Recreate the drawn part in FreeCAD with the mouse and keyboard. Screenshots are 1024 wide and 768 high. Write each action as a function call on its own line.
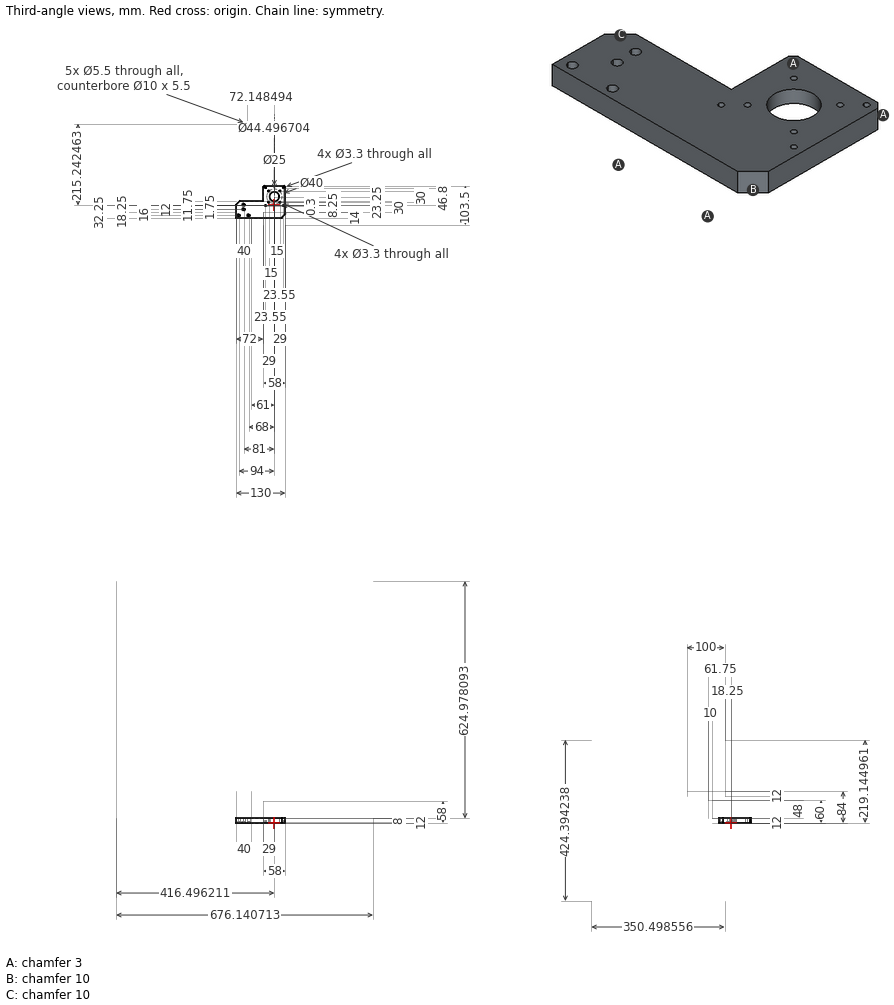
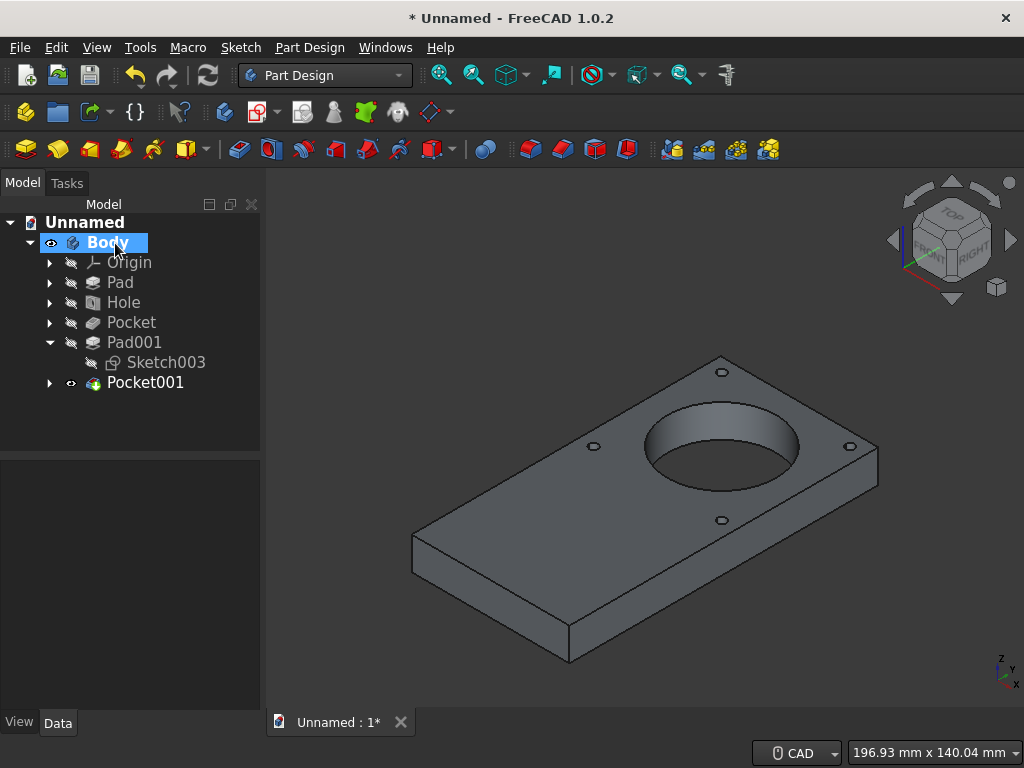
click(569, 644)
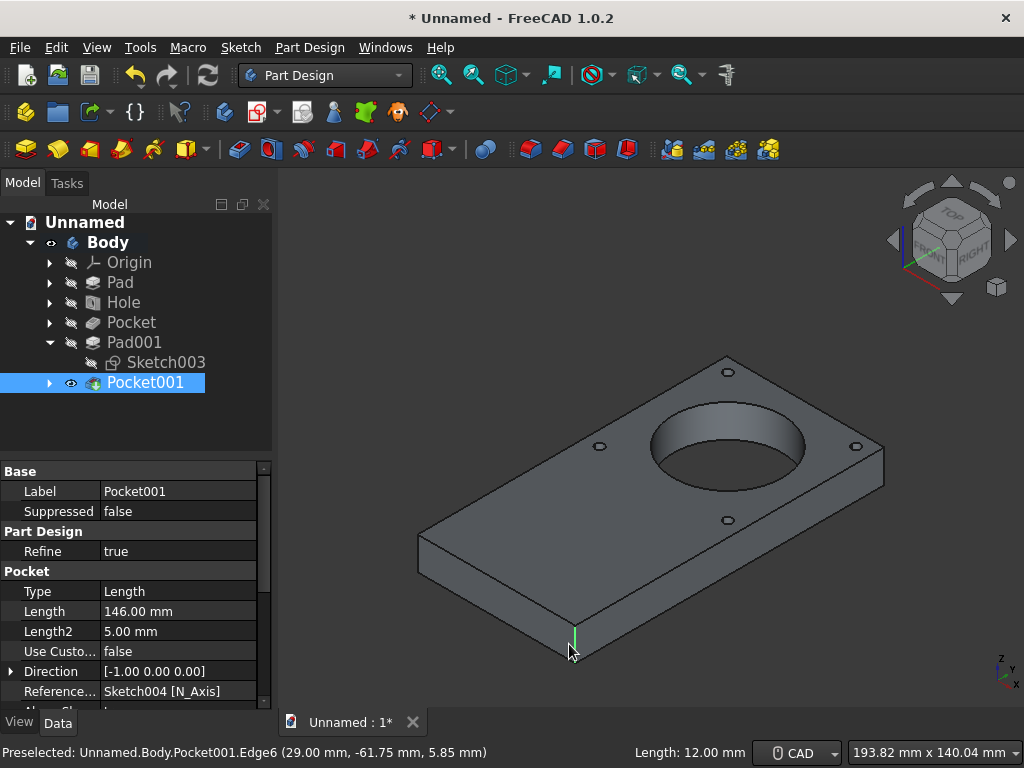
key(2)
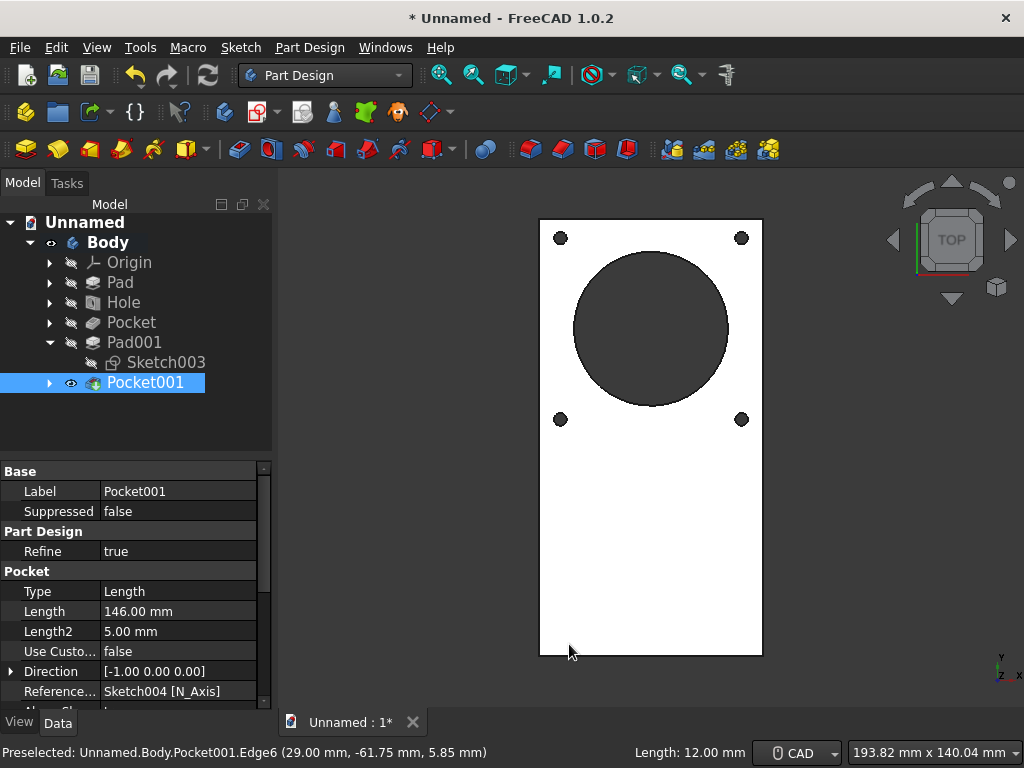
key(0)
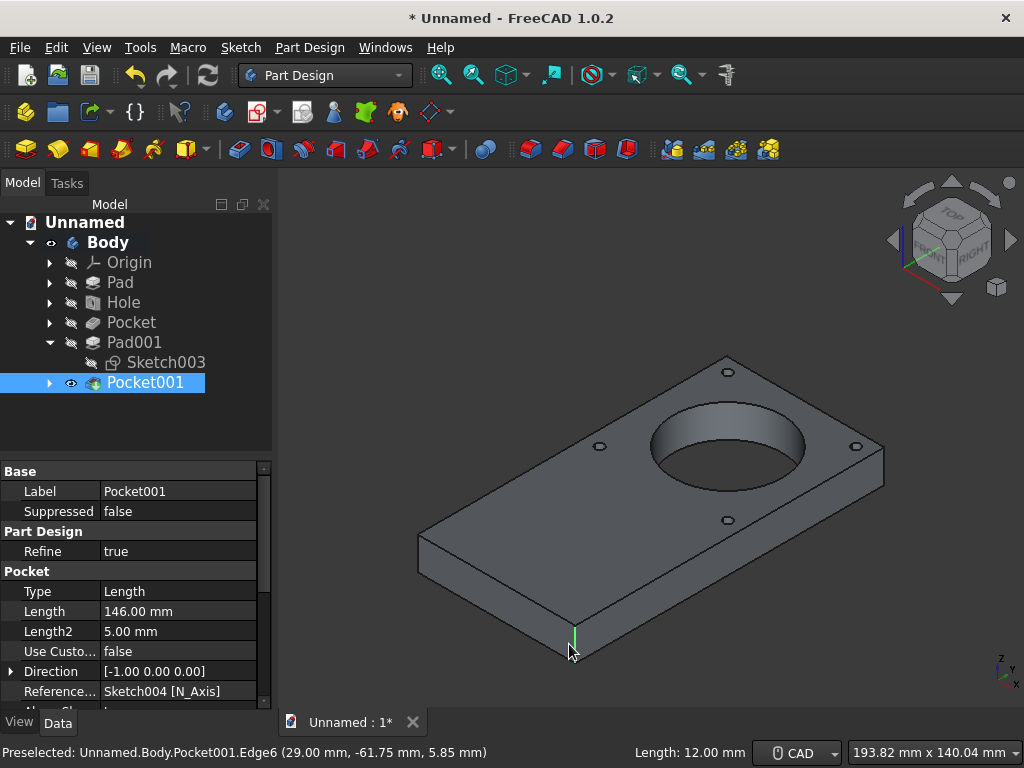
key(1)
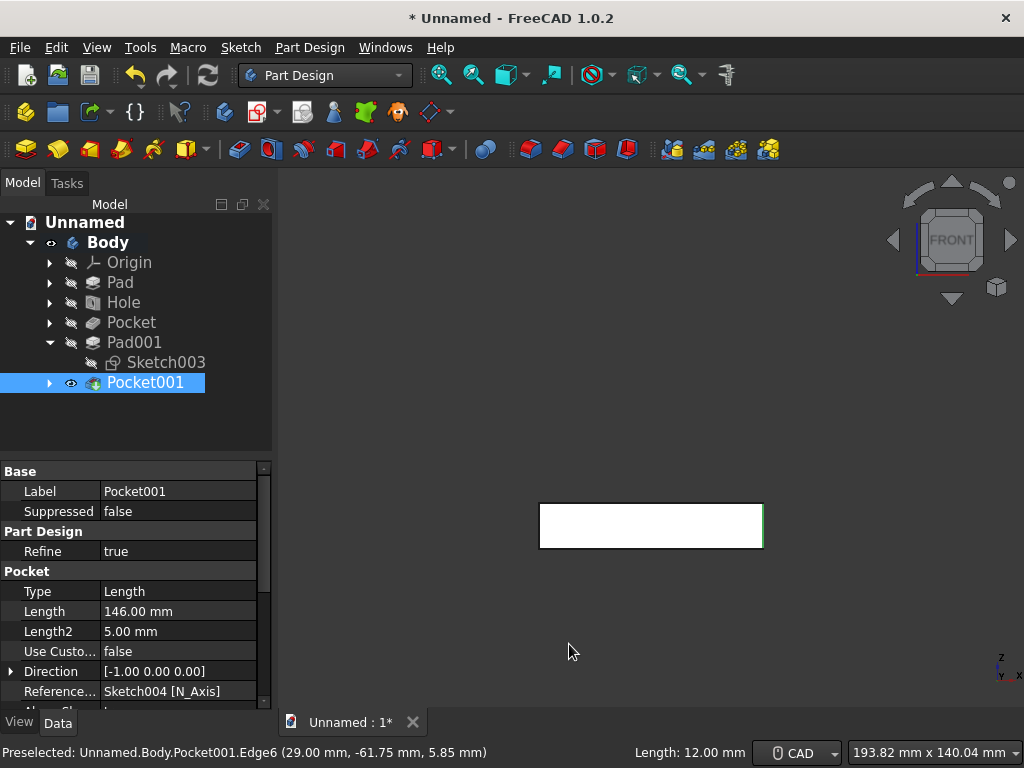
click(442, 76)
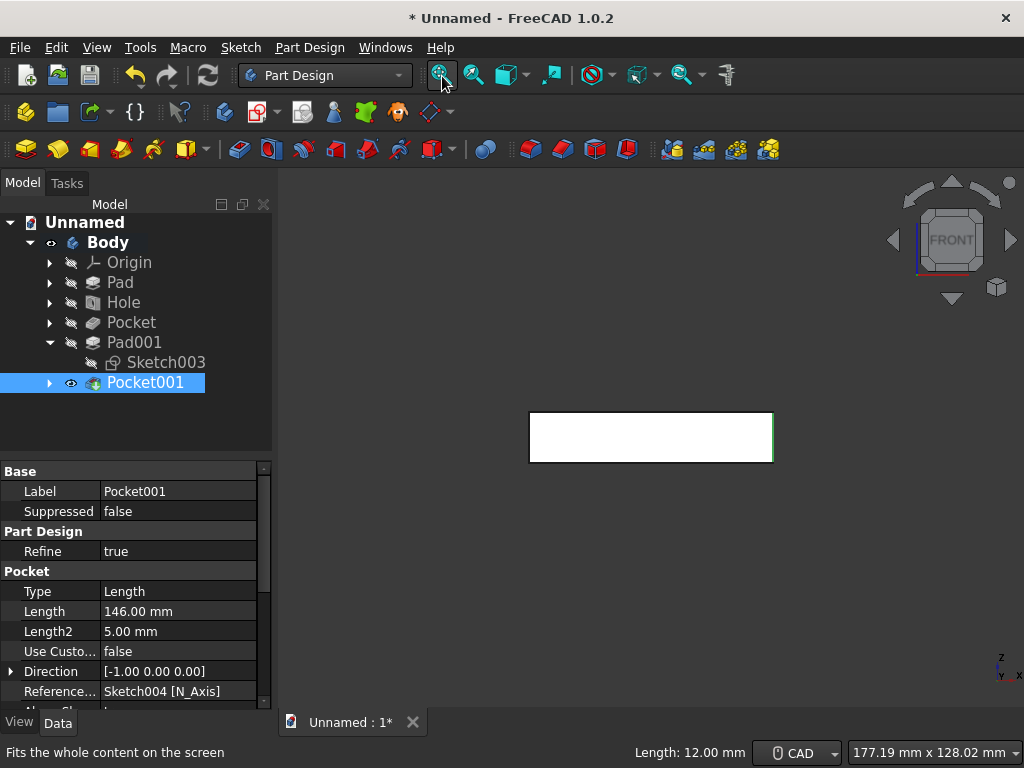
click(529, 437, ctrl)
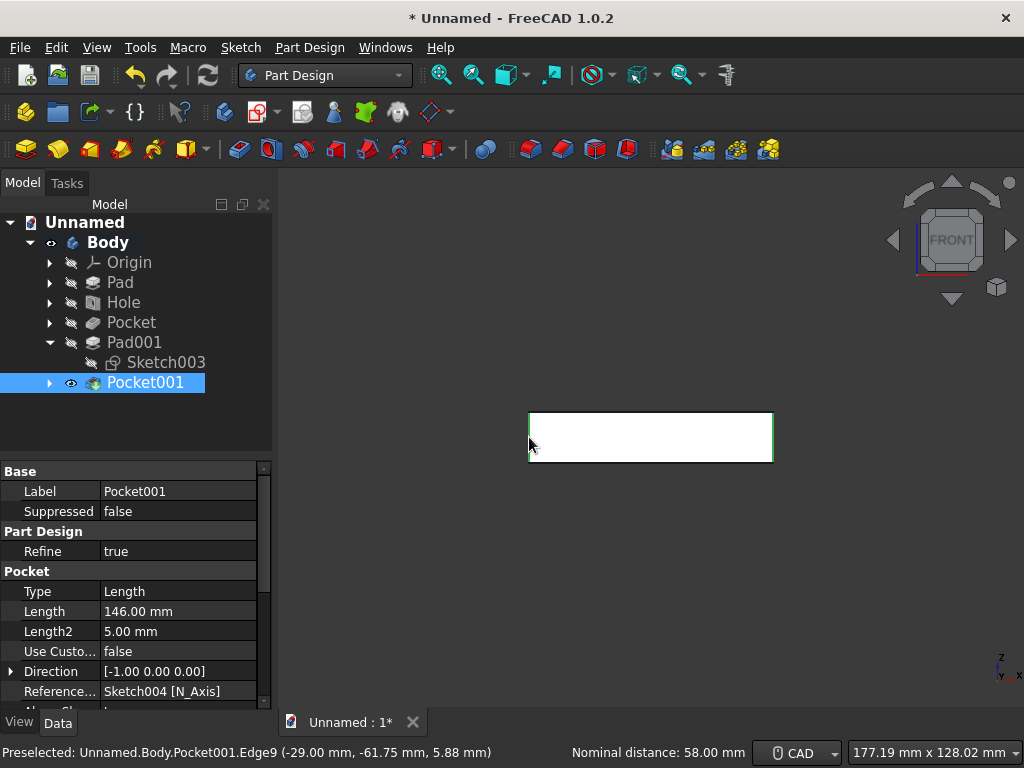
key(3)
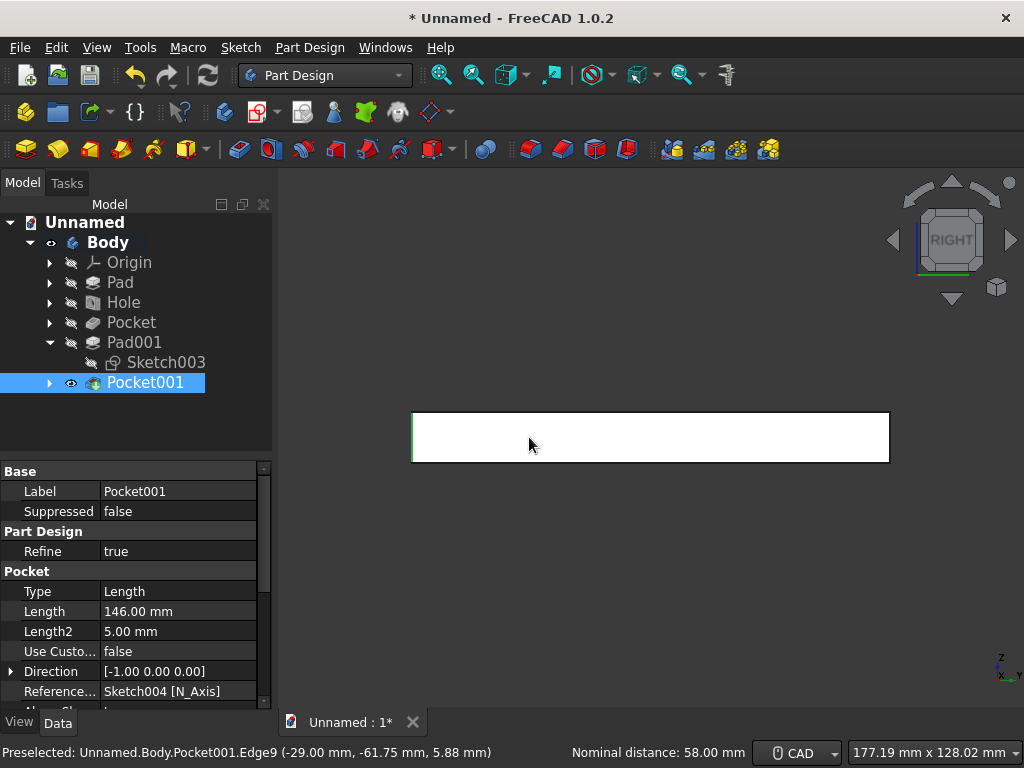
click(890, 436, ctrl)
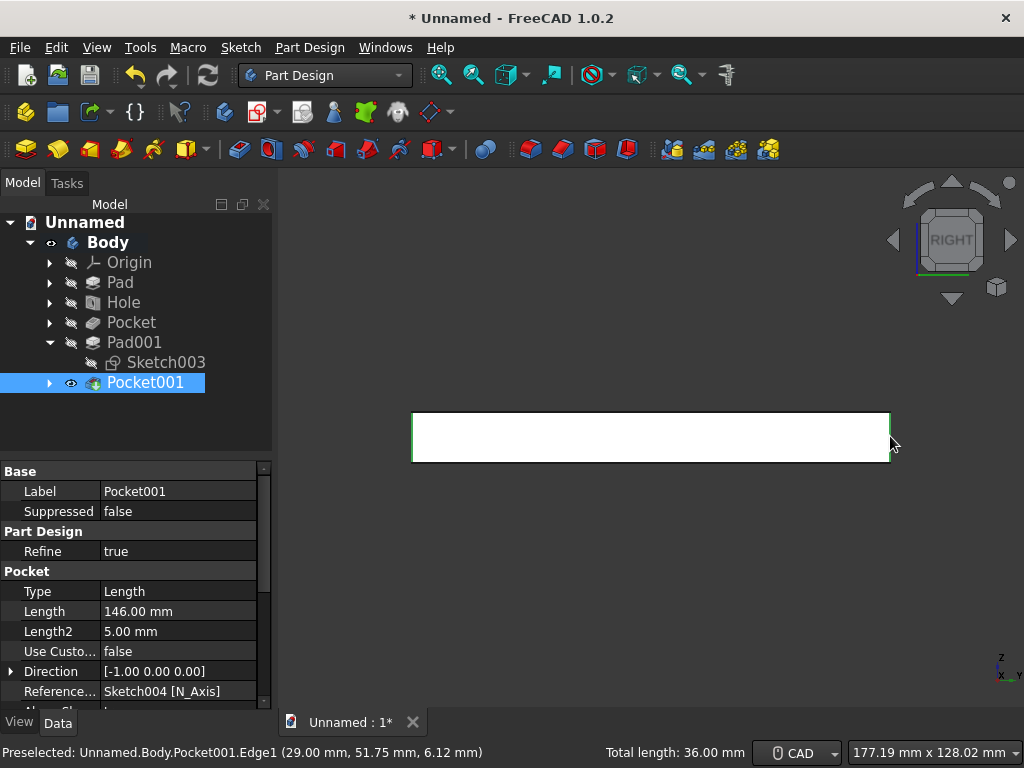
key(5)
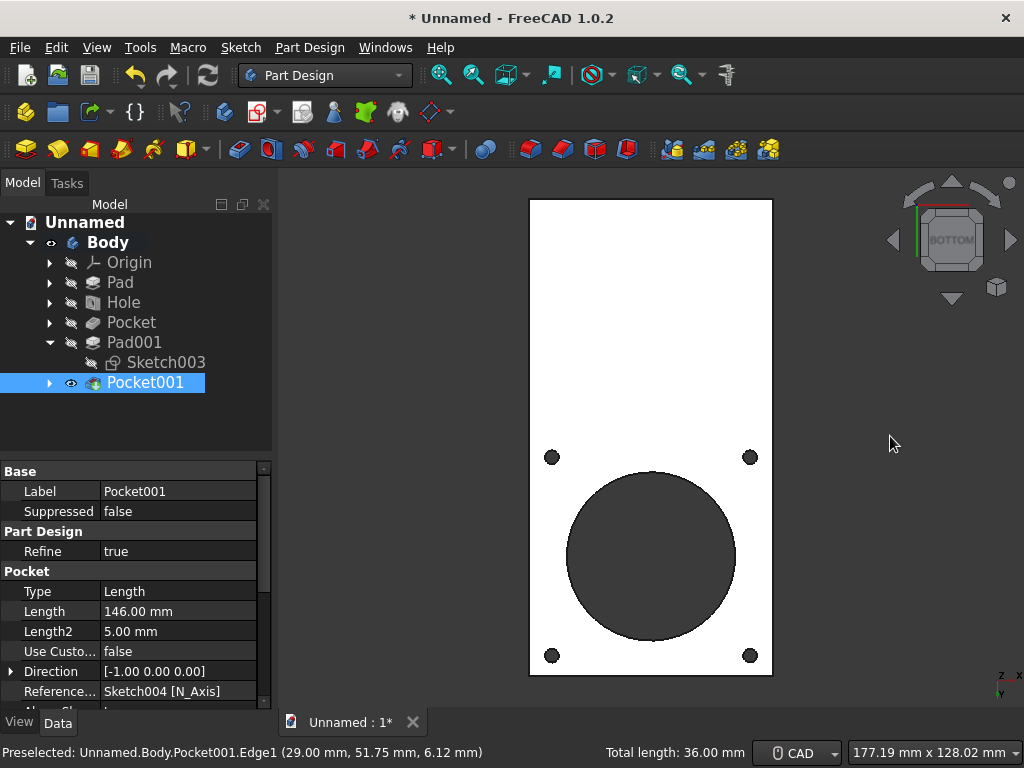
key(4)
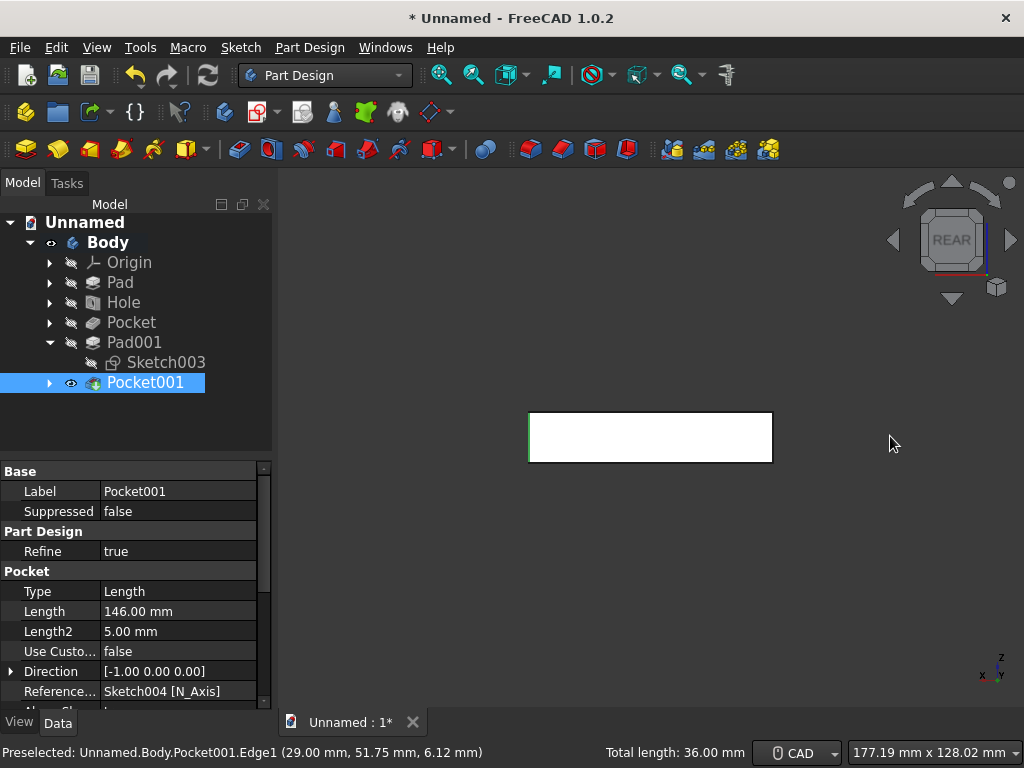
click(442, 76)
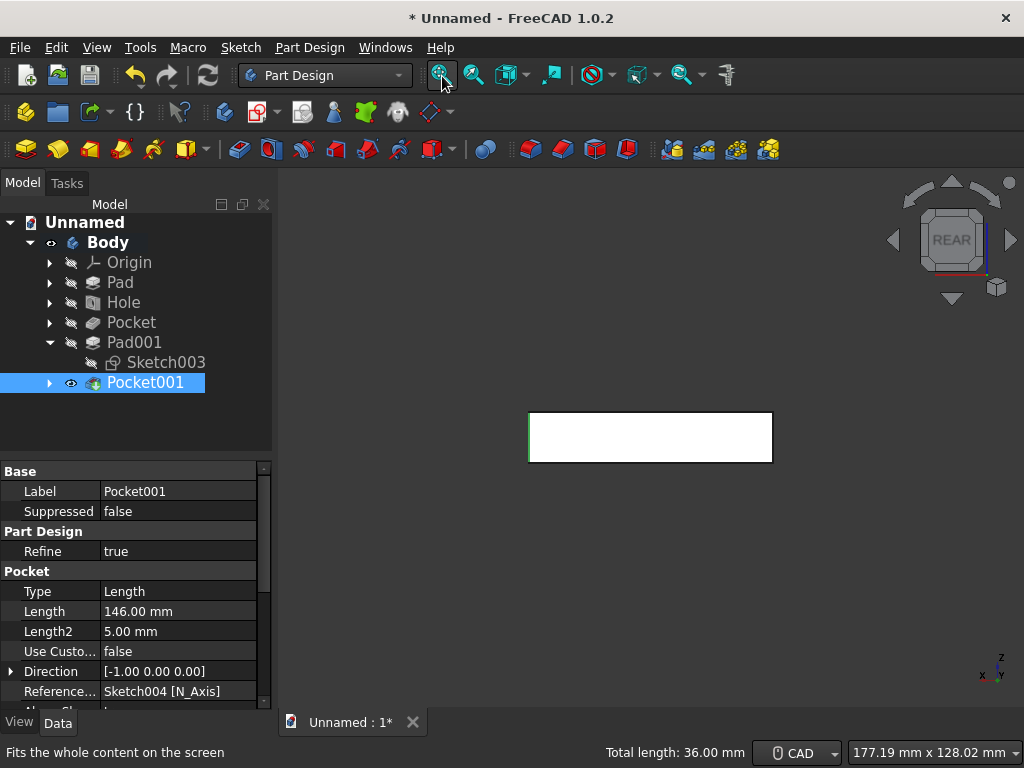
click(773, 437, ctrl)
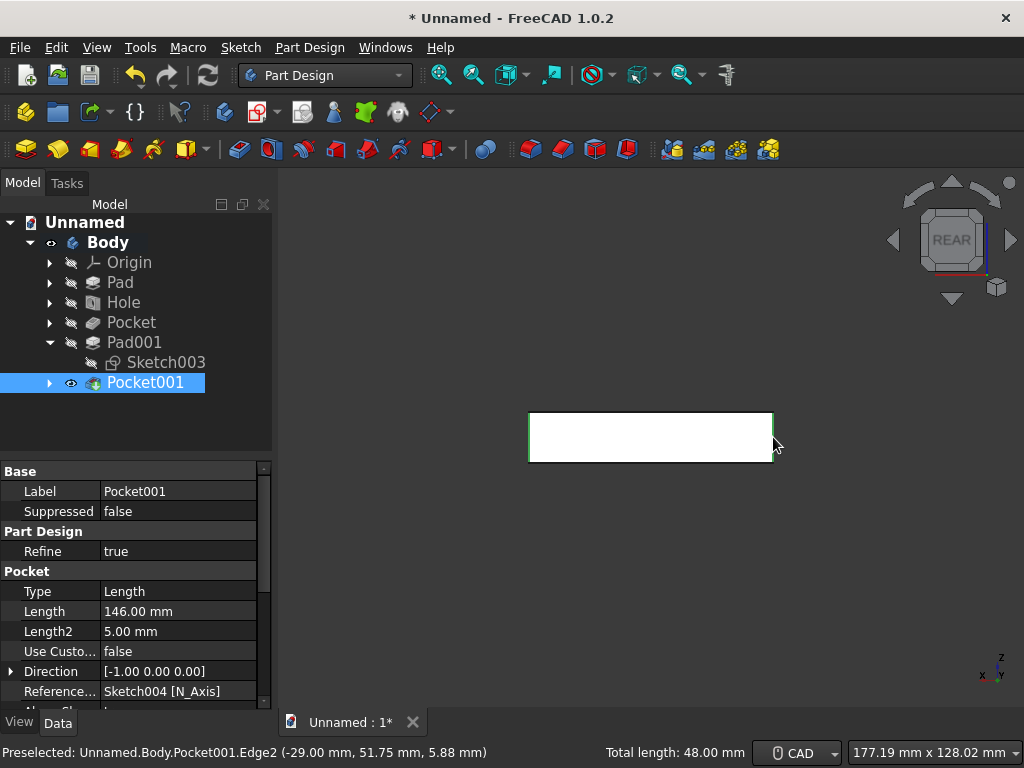
click(564, 150)